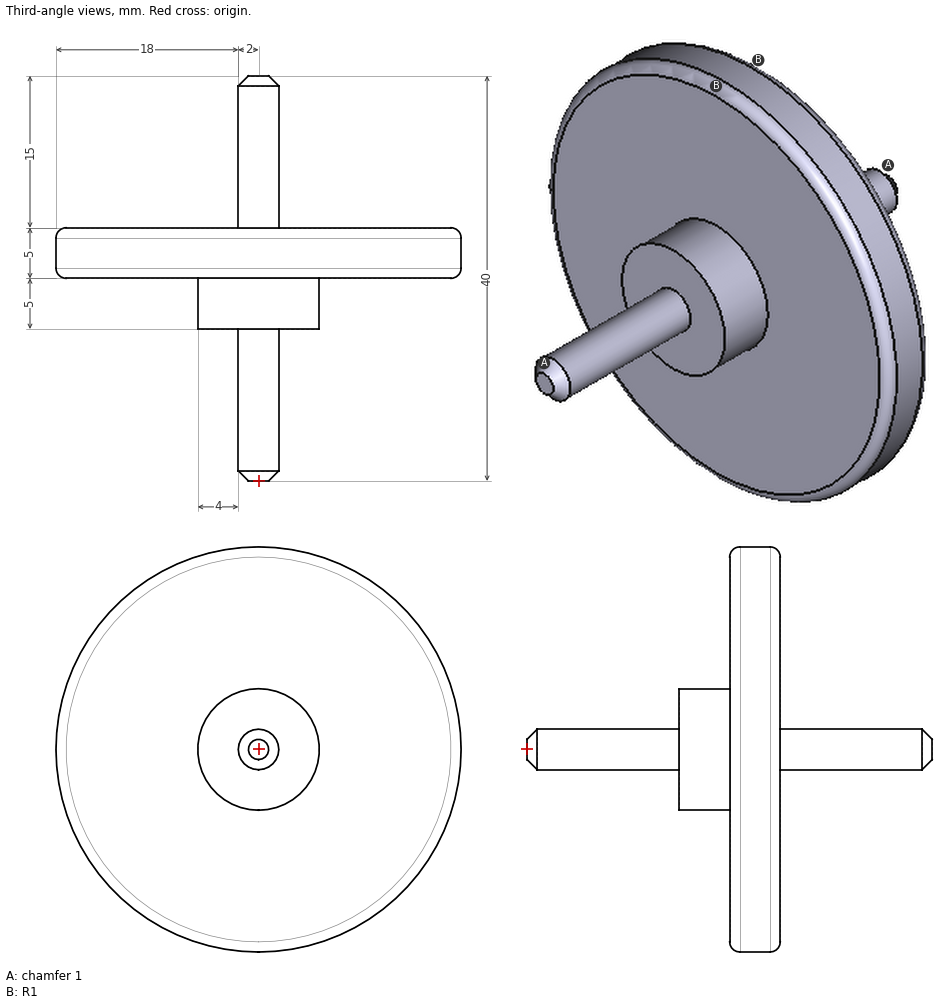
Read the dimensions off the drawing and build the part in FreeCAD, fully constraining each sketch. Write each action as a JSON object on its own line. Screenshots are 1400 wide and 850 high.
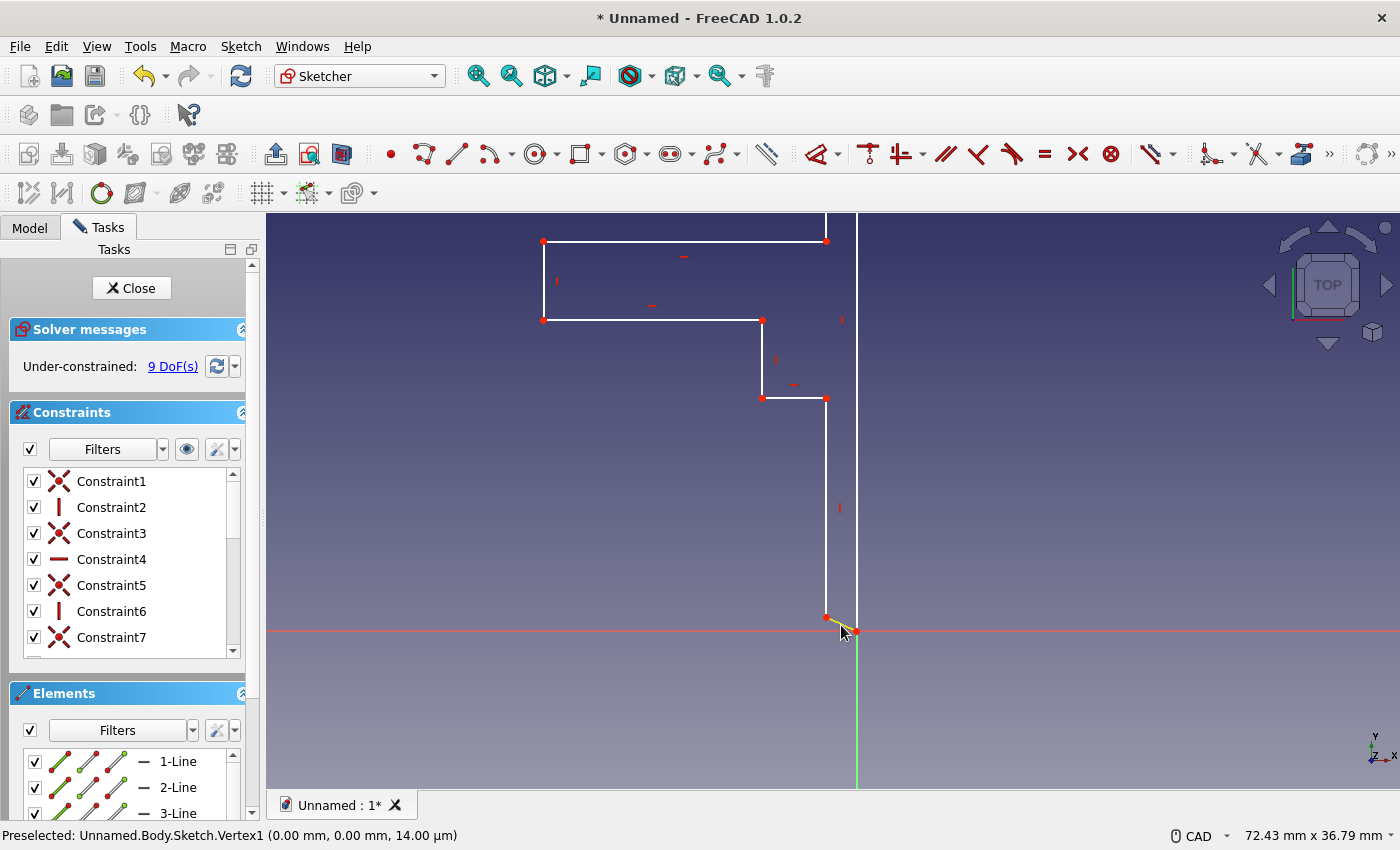
{"action": "left_click", "coordinate": [841, 624]}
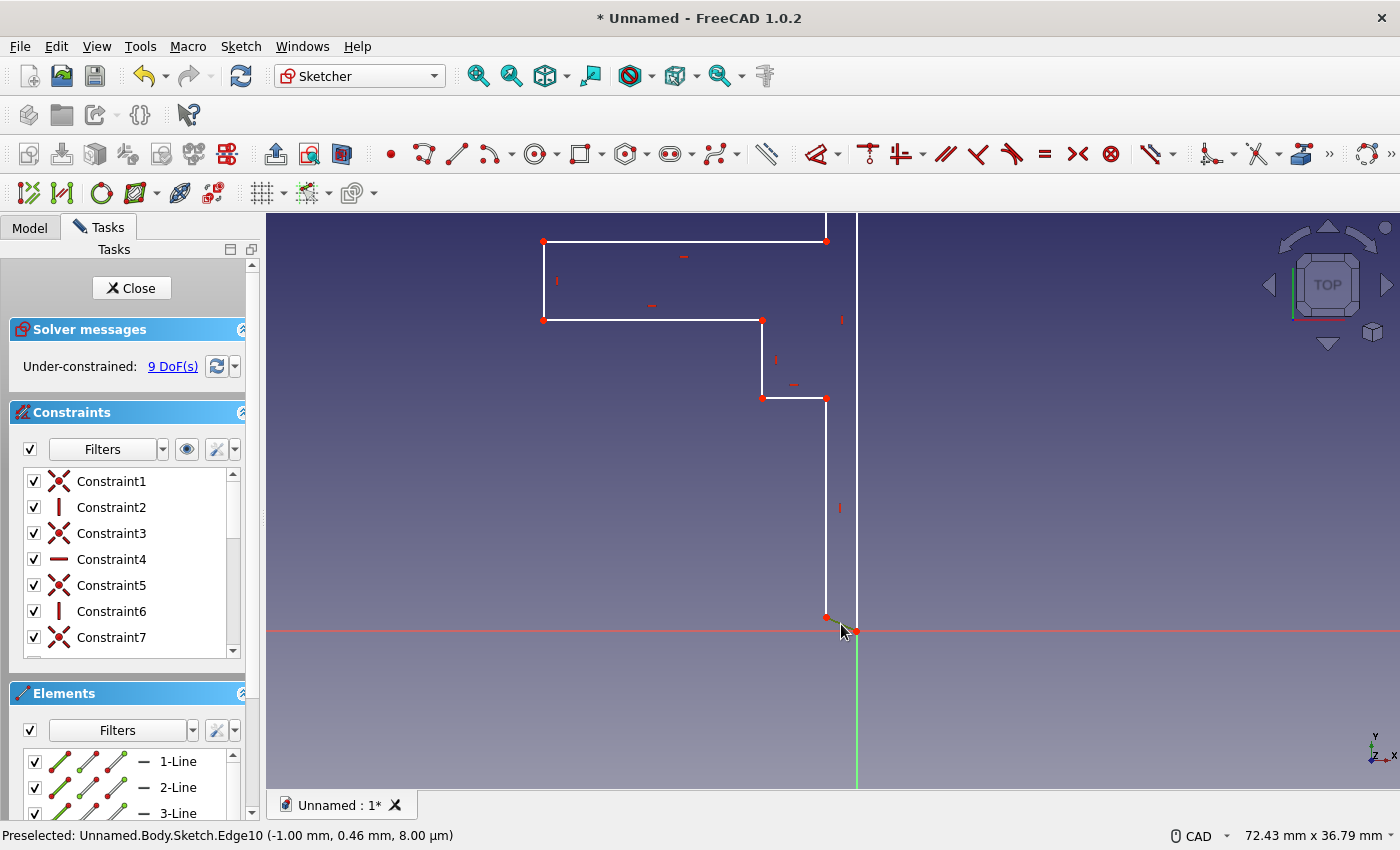
{"action": "left_click", "coordinate": [922, 154]}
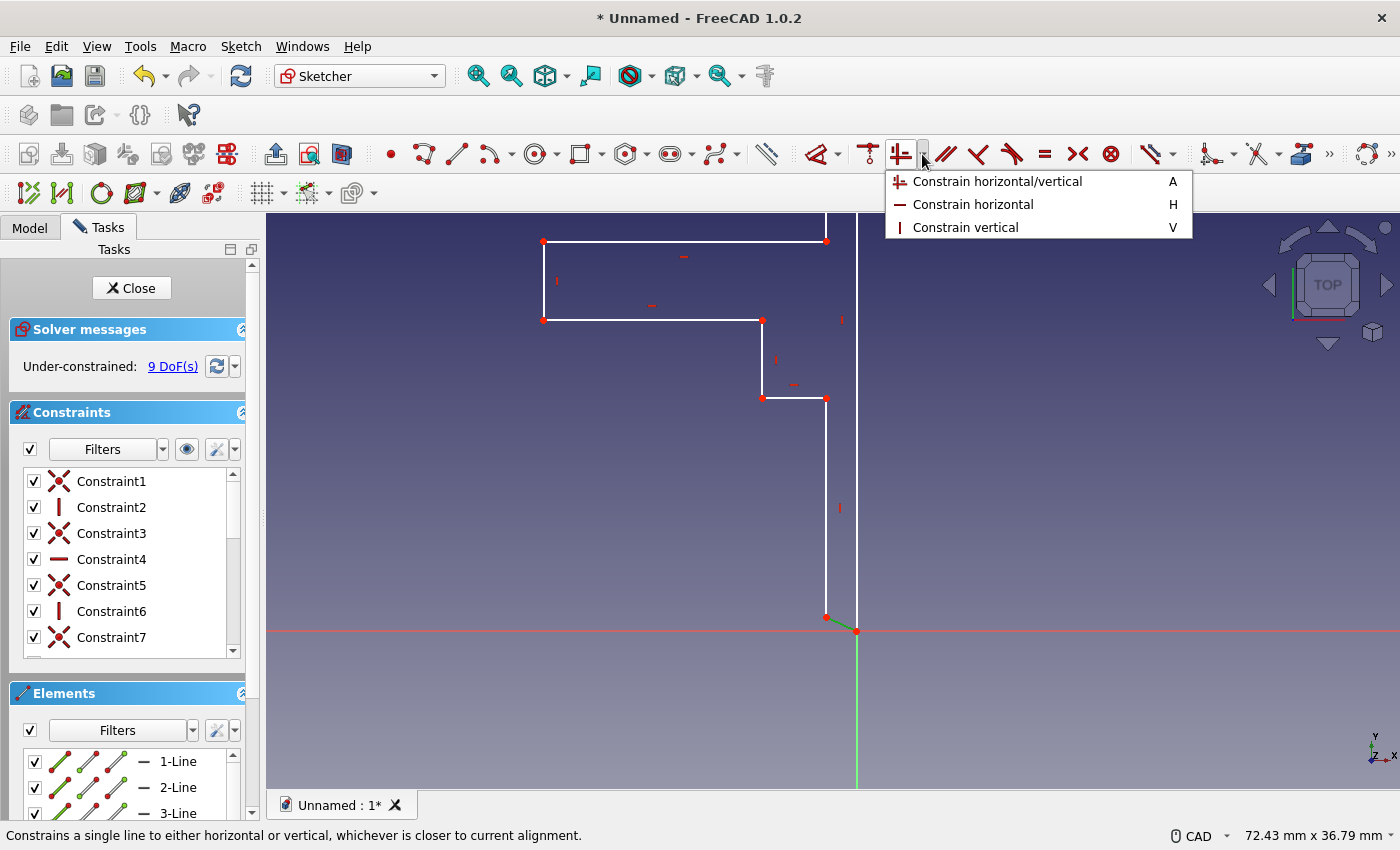
{"action": "left_click", "coordinate": [1039, 204]}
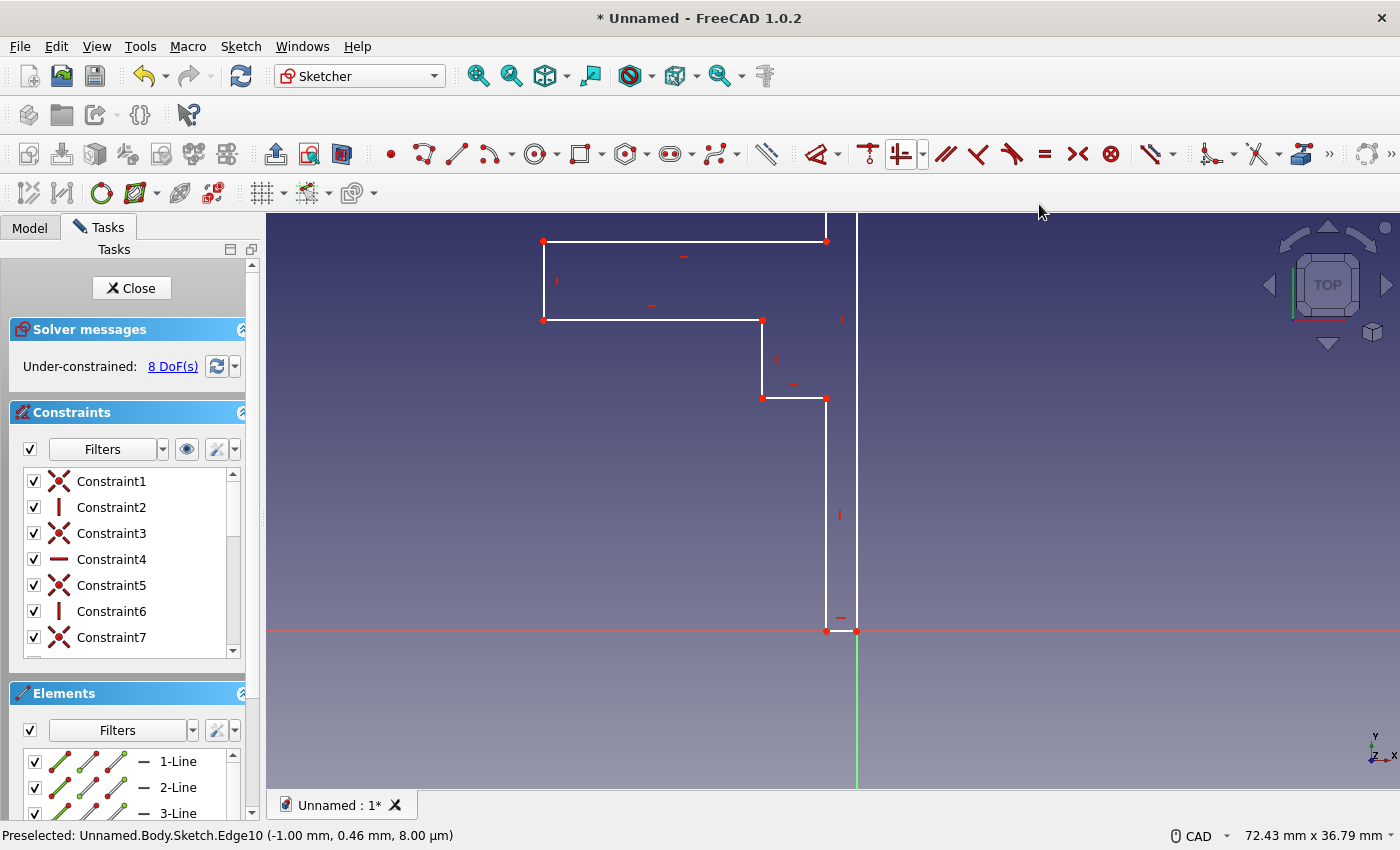
{"action": "key", "text": "d"}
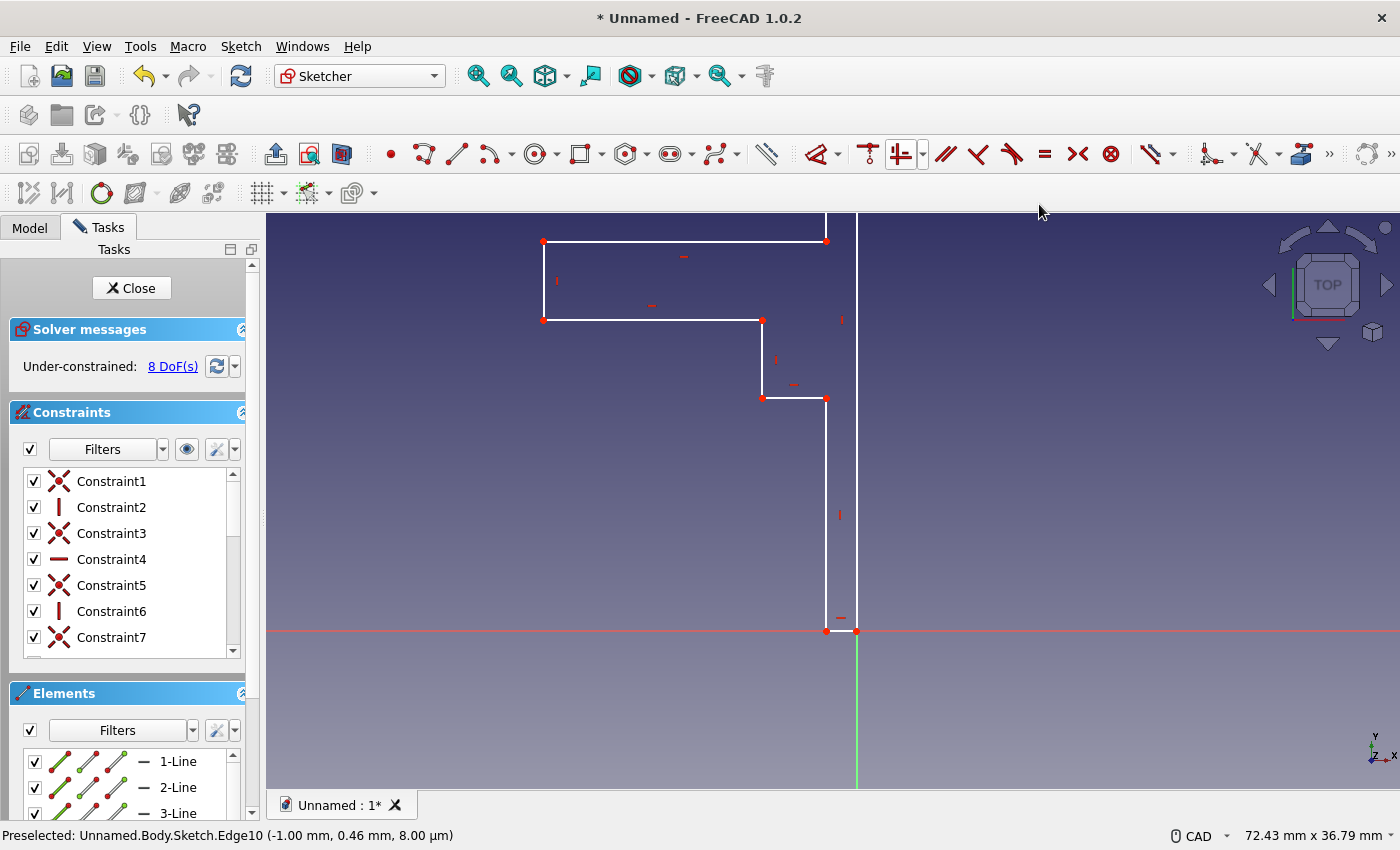
{"action": "scroll", "coordinate": [842, 723], "scroll_direction": "down", "scroll_amount": 3}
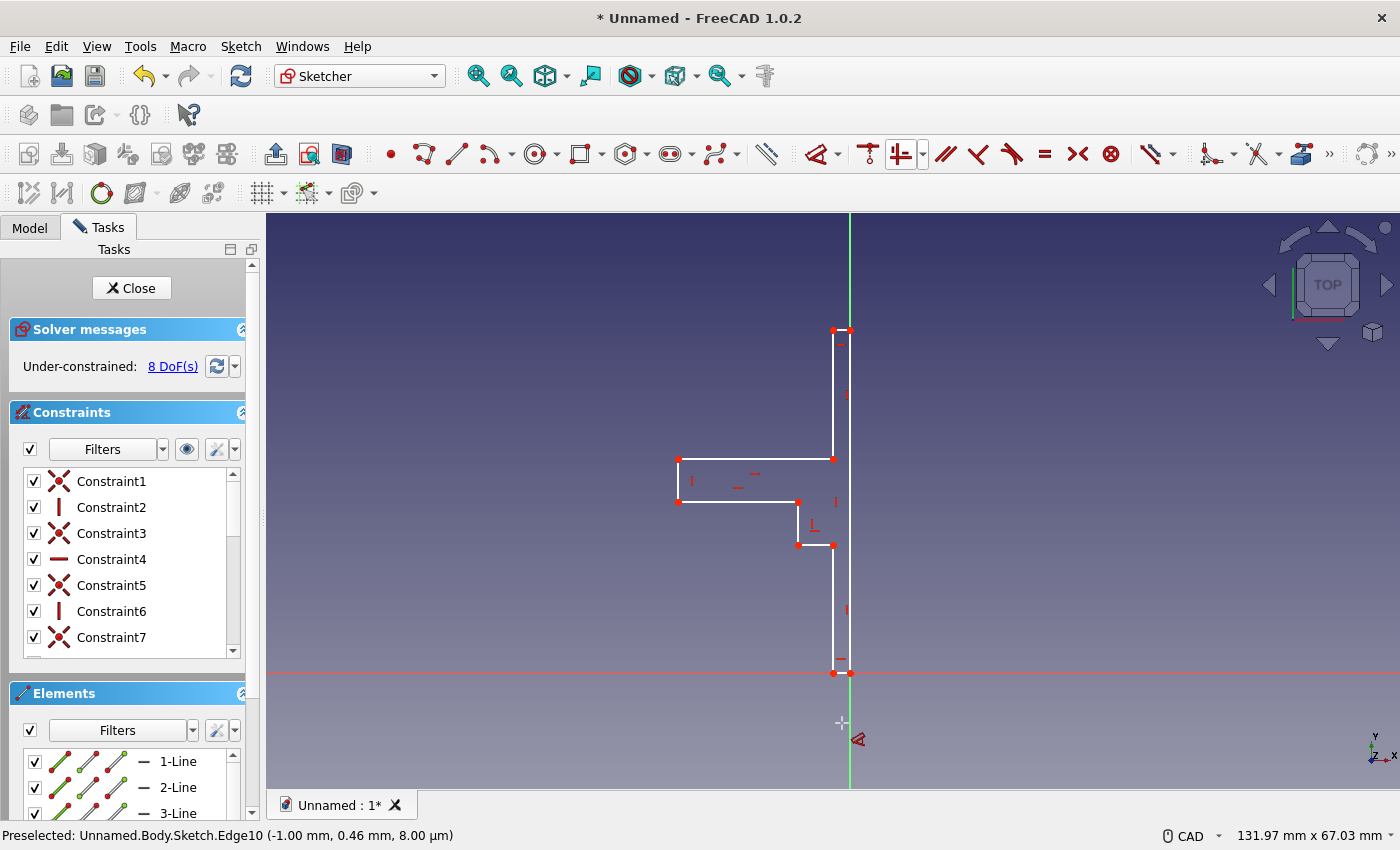
{"action": "scroll", "coordinate": [845, 330], "scroll_direction": "up", "scroll_amount": 5}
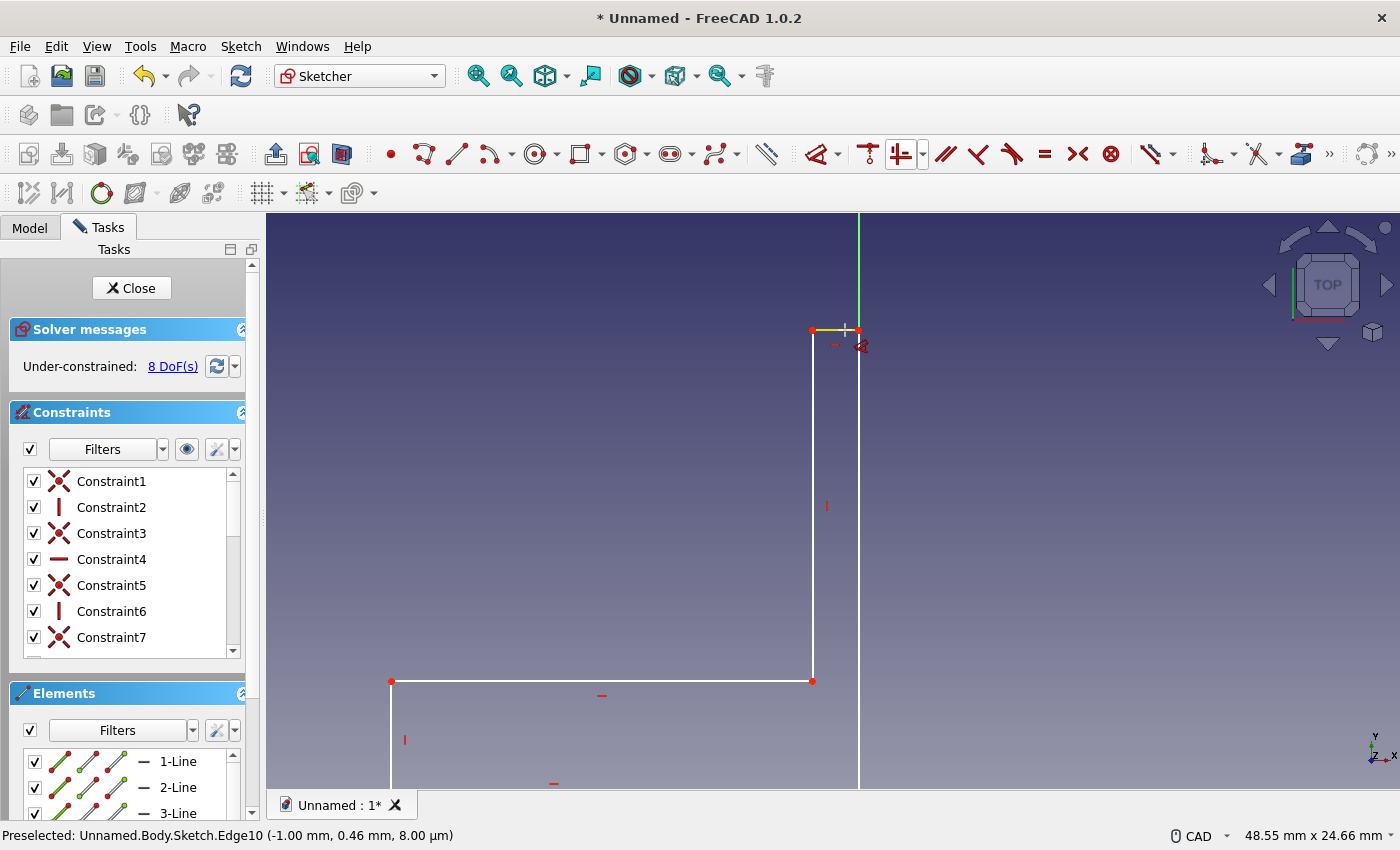
{"action": "left_click", "coordinate": [845, 330]}
{"action": "left_click", "coordinate": [836, 296]}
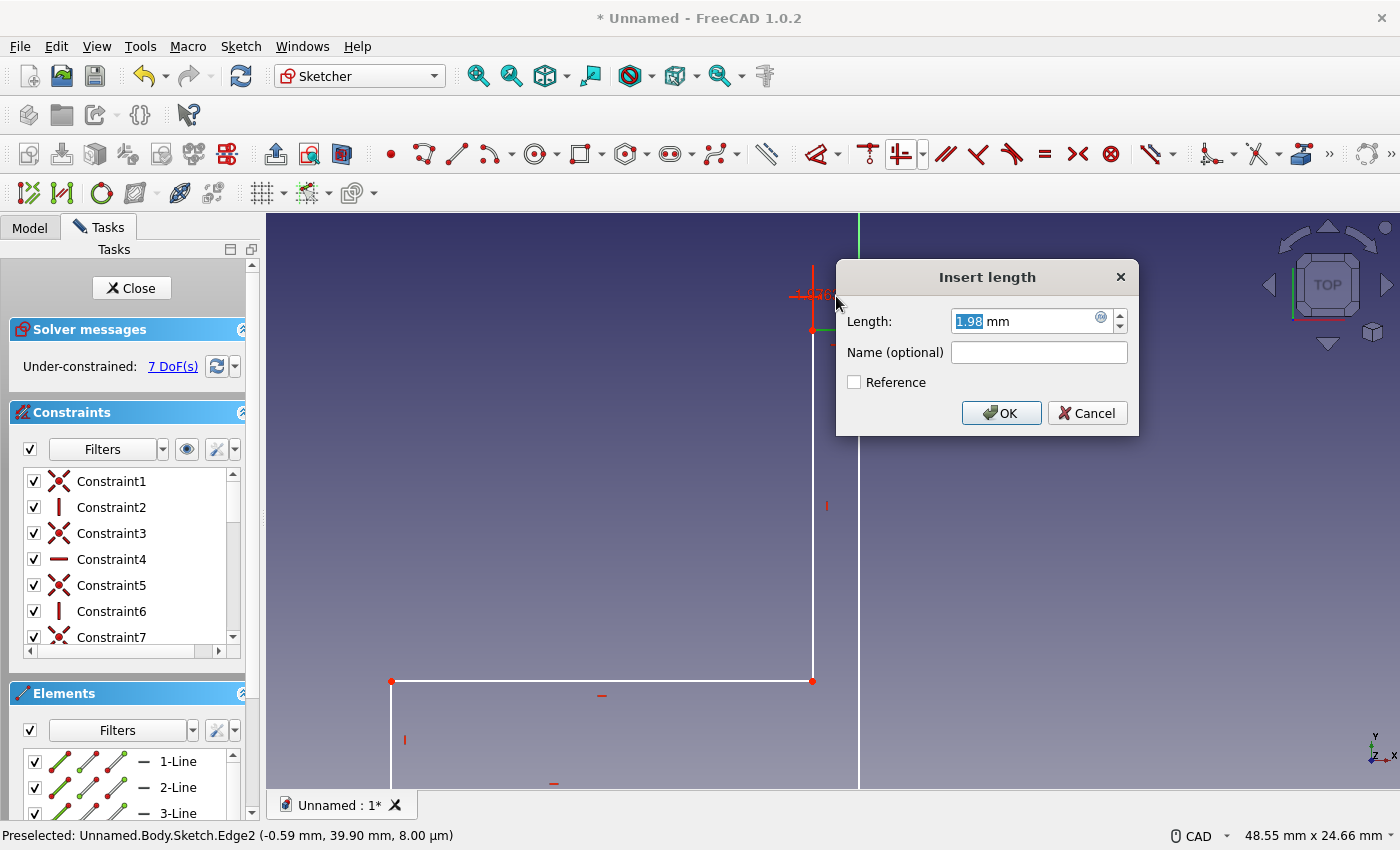
{"action": "type", "text": "2"}
{"action": "key", "text": "Return"}